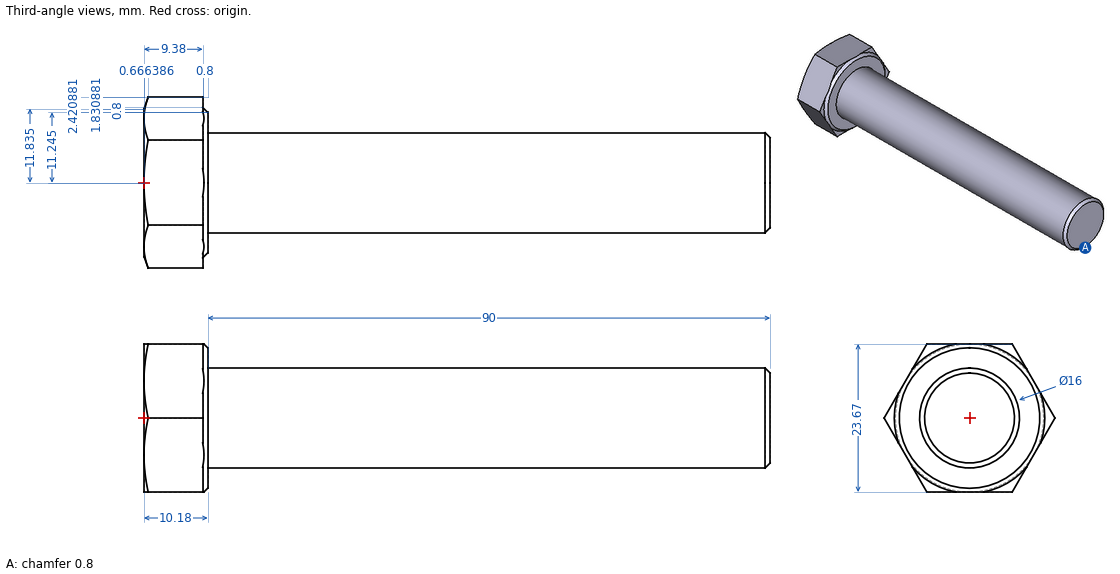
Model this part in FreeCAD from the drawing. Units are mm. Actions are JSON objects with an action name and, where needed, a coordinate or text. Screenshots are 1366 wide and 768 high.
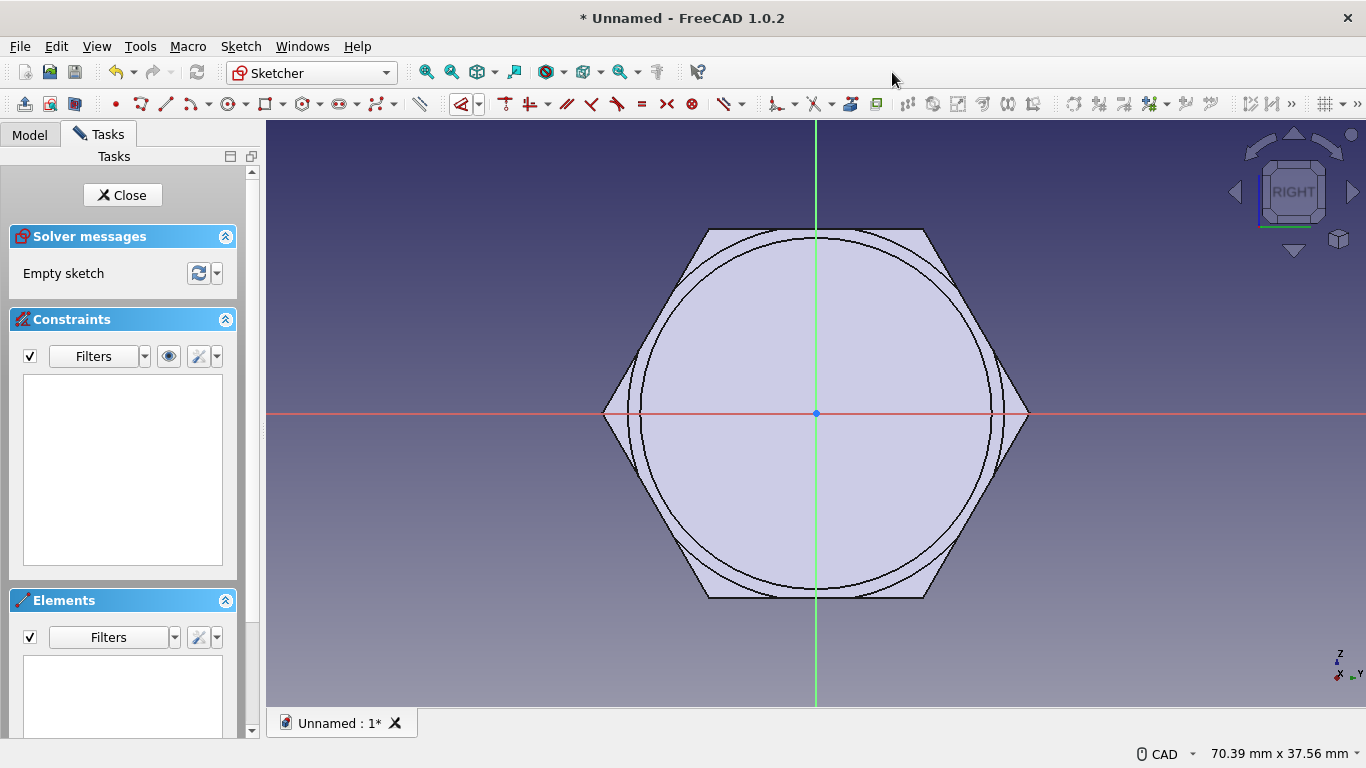
{"action": "scroll", "coordinate": [955, 413], "scroll_direction": "up", "scroll_amount": 2}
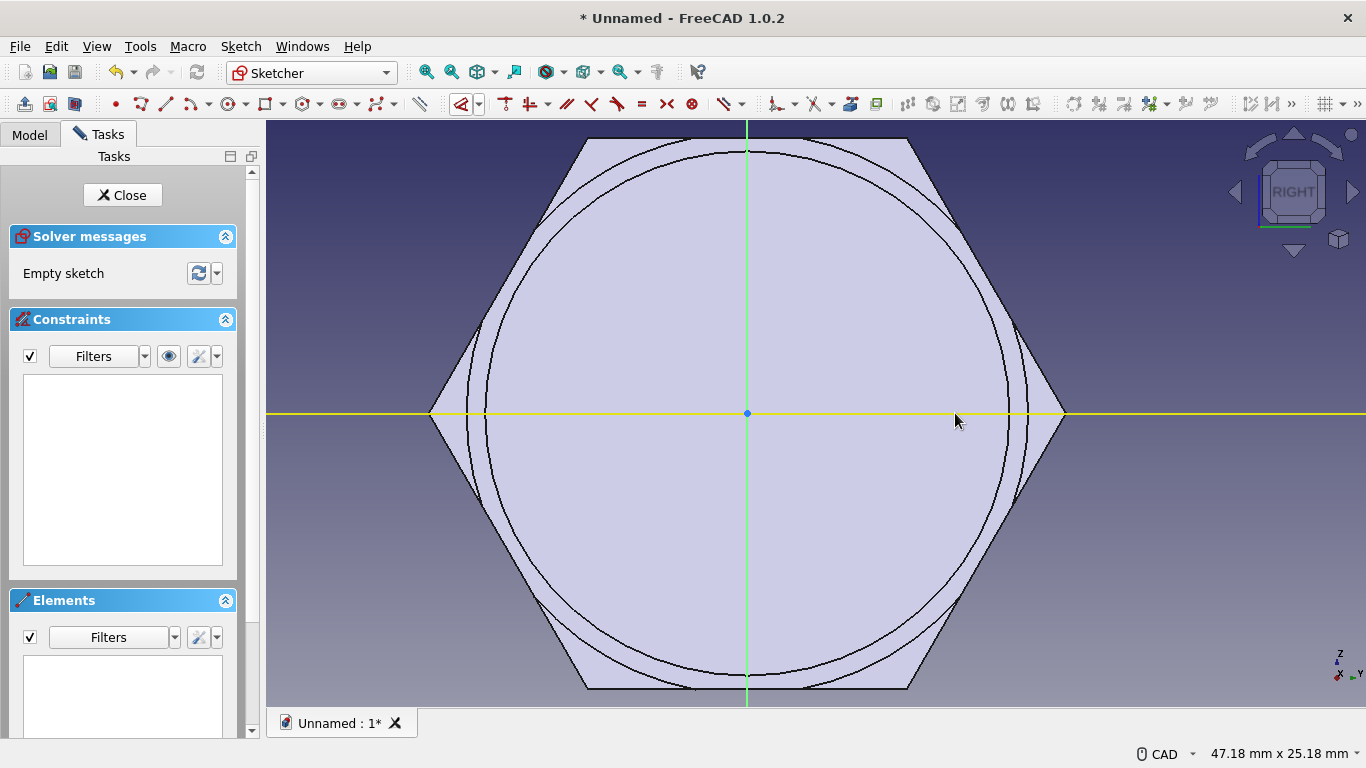
{"action": "key", "text": "g c"}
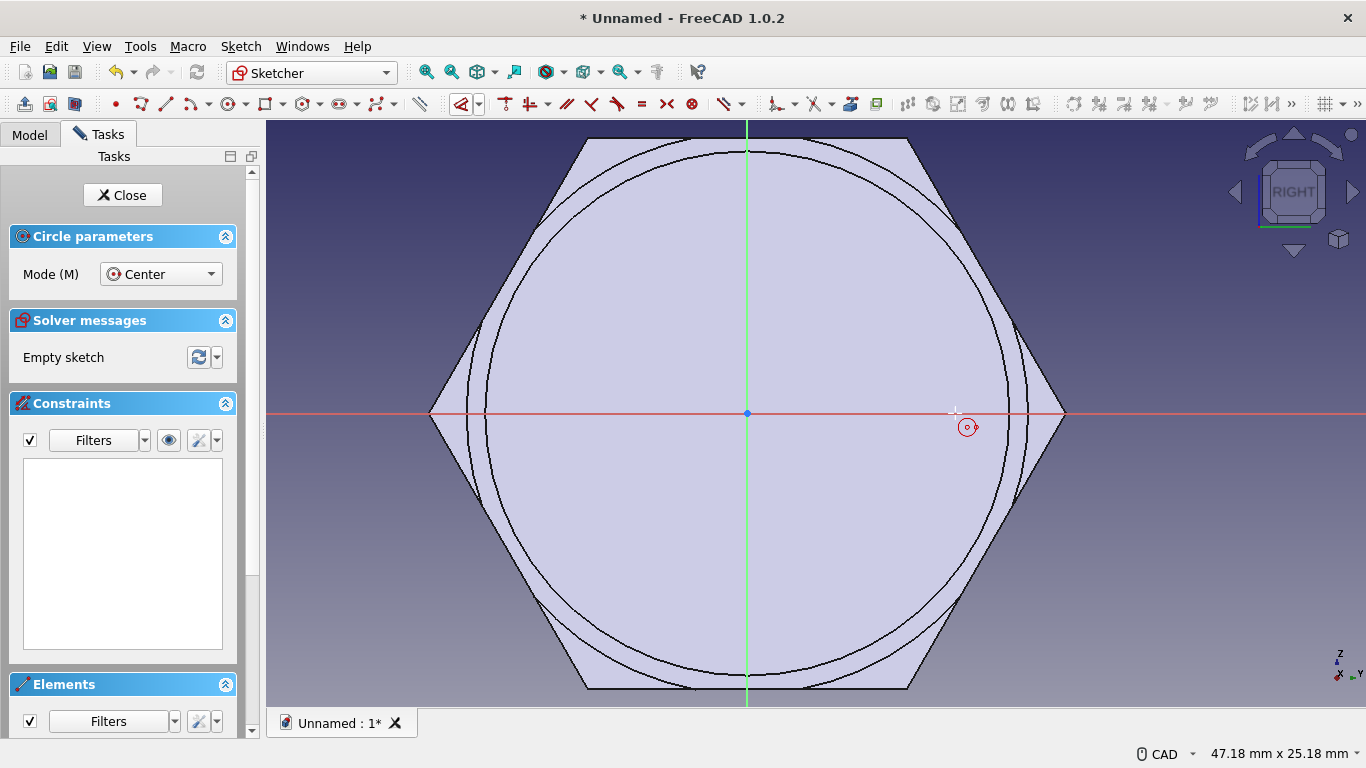
{"action": "left_click", "coordinate": [747, 413]}
{"action": "left_click", "coordinate": [879, 282]}
{"action": "key", "text": "Escape"}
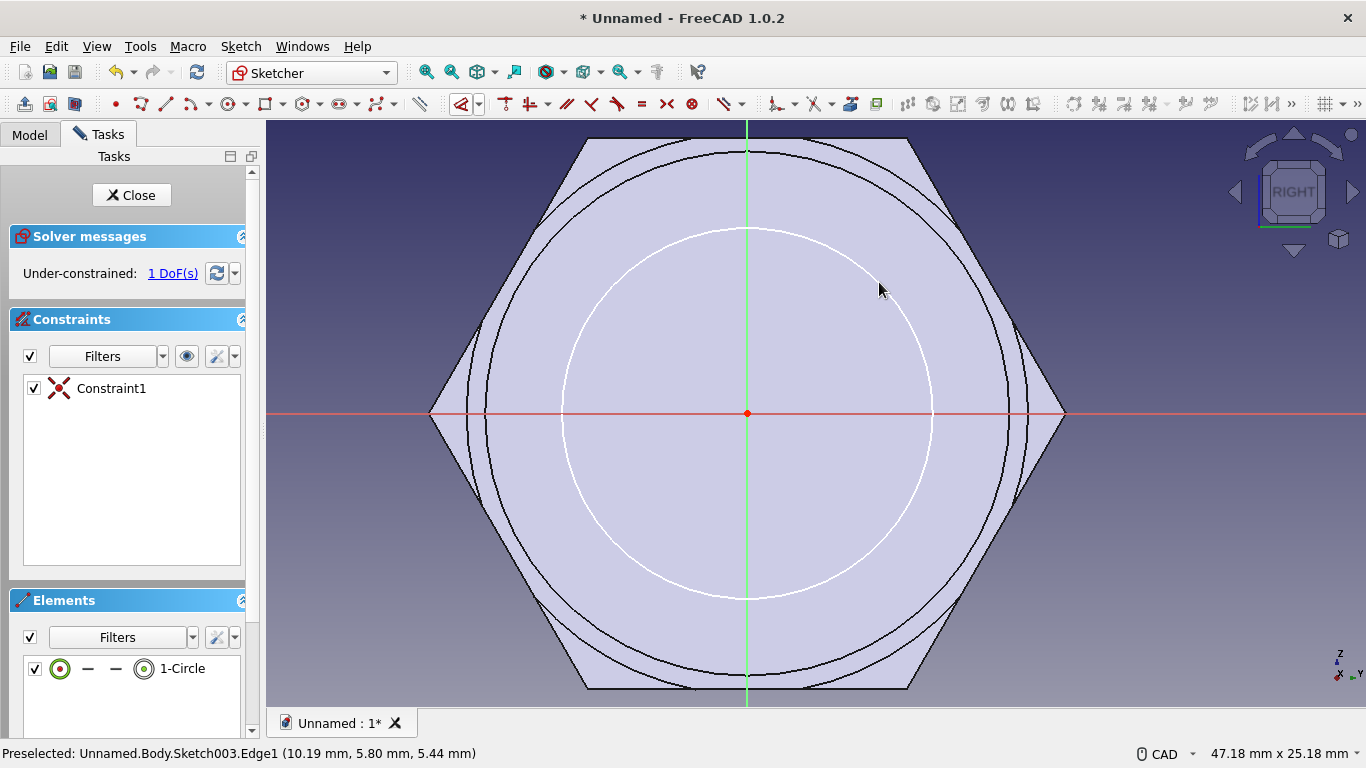
{"action": "left_click", "coordinate": [878, 282]}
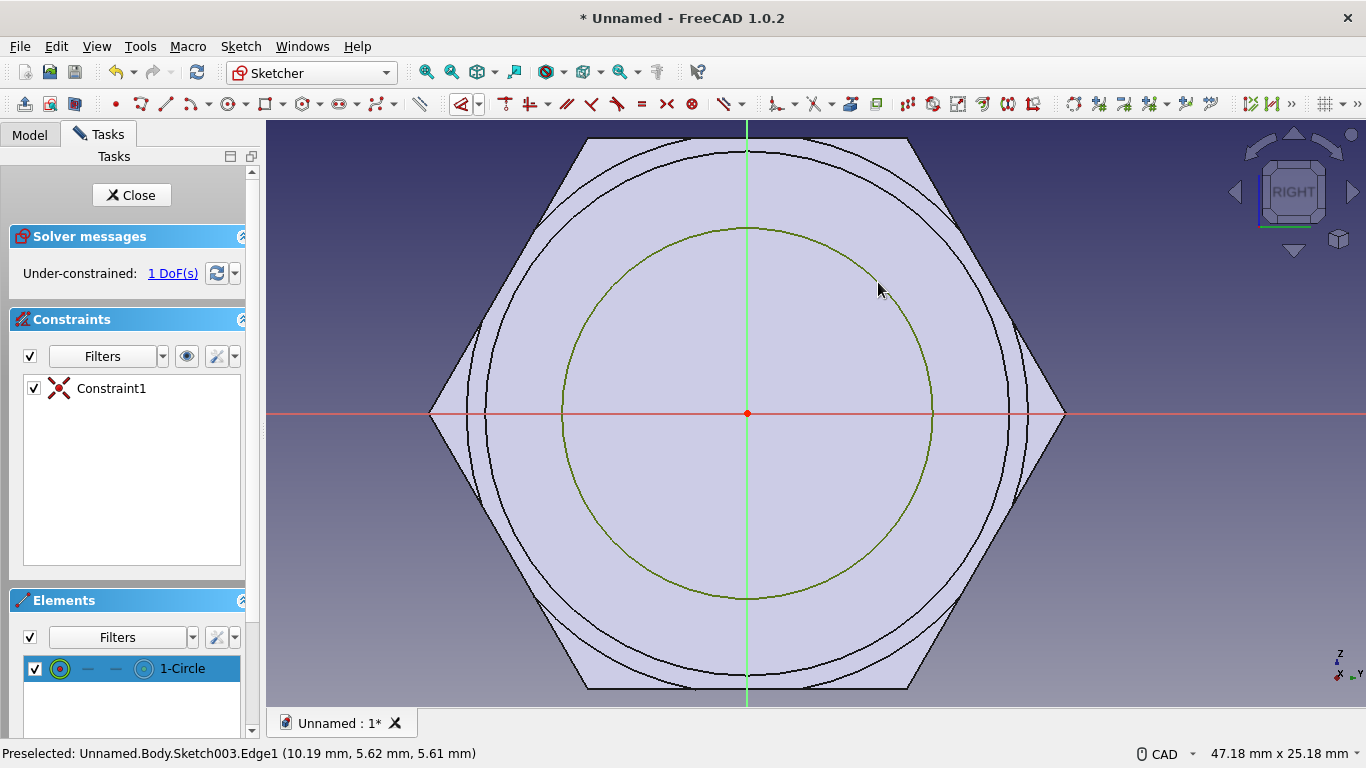
{"action": "key", "text": "k o"}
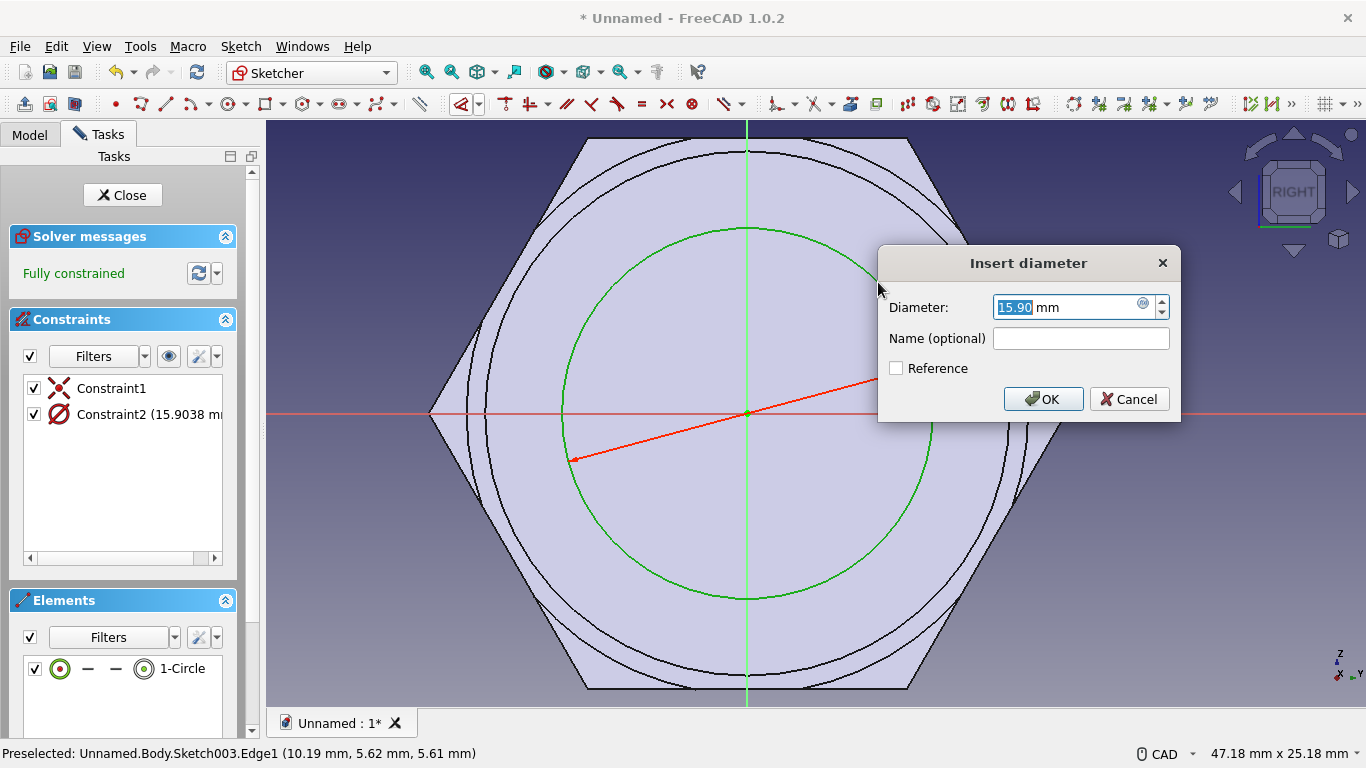
{"action": "type", "text": "16"}
{"action": "key", "text": "Return"}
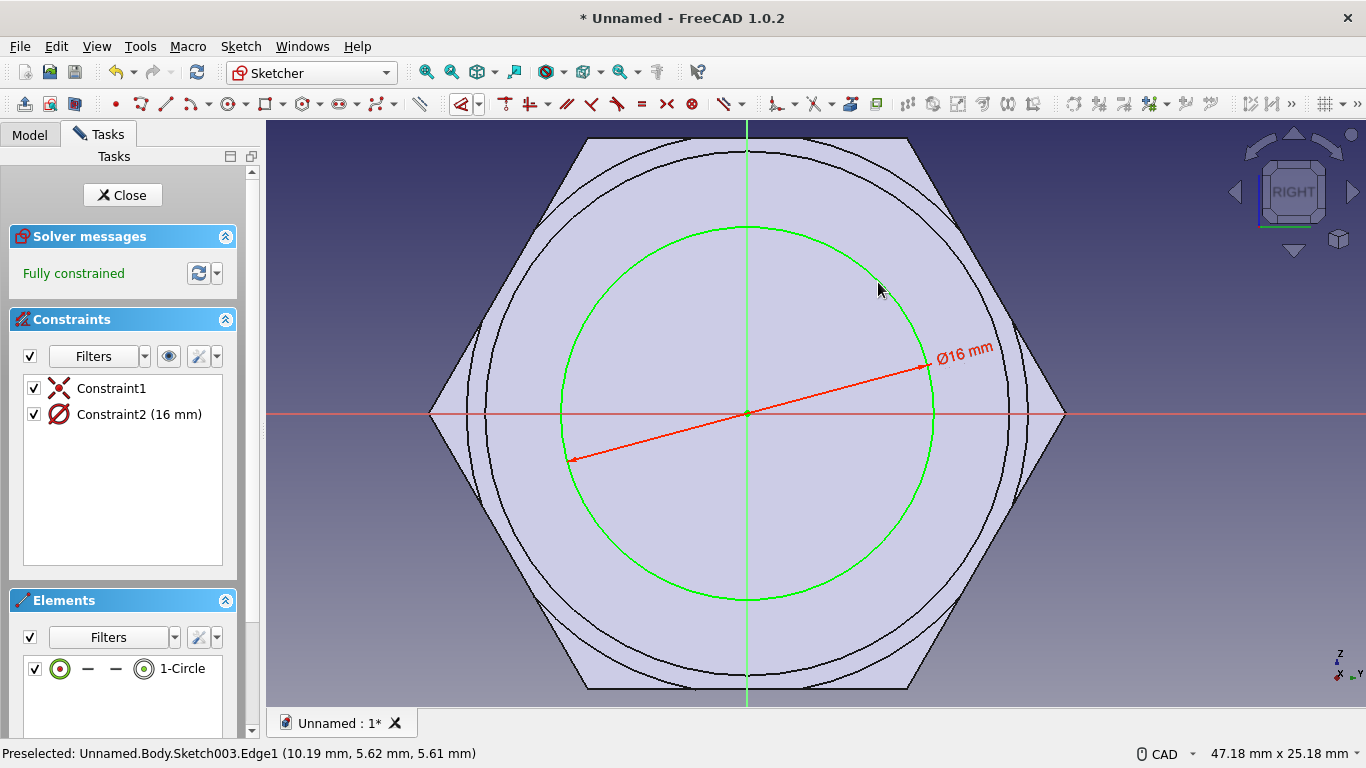
{"action": "left_click", "coordinate": [123, 195]}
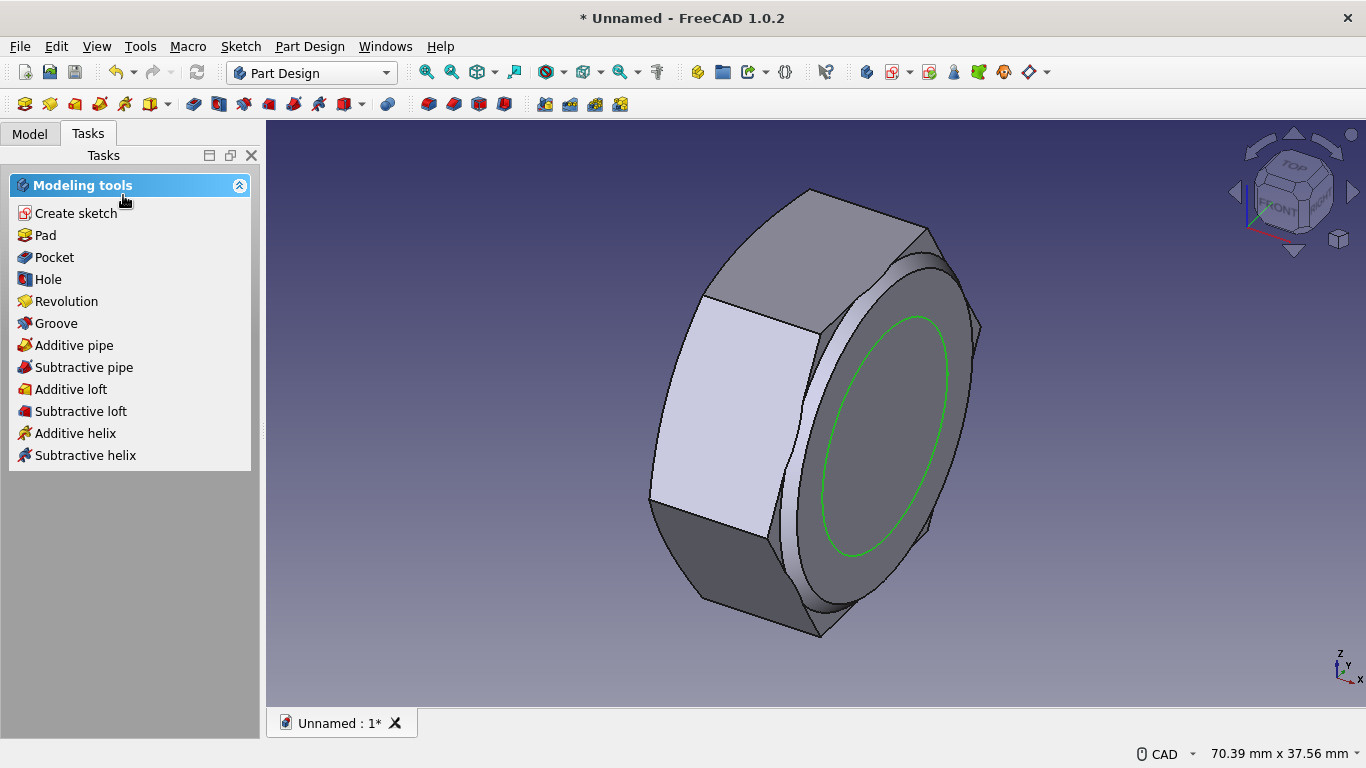
{"action": "left_click", "coordinate": [25, 104]}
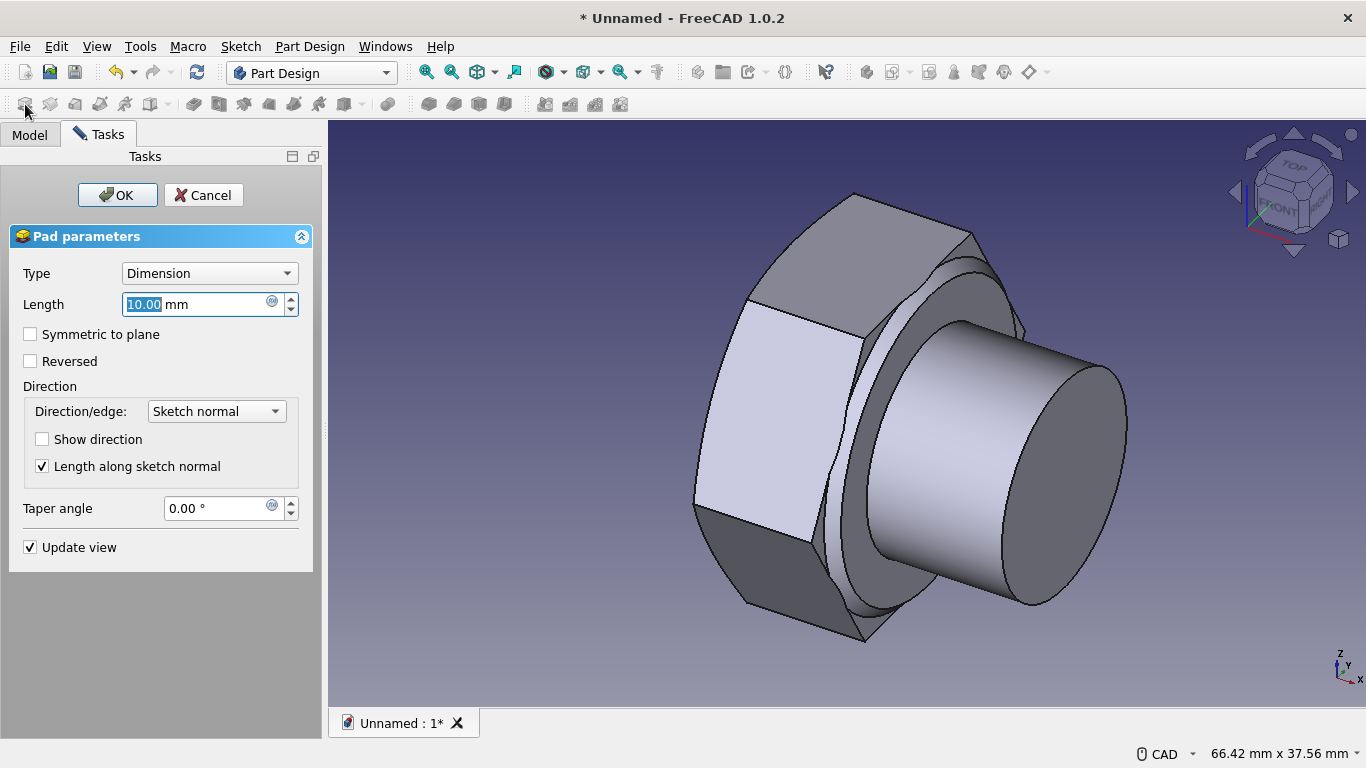
{"action": "type", "text": "90"}
{"action": "key", "text": "Tab"}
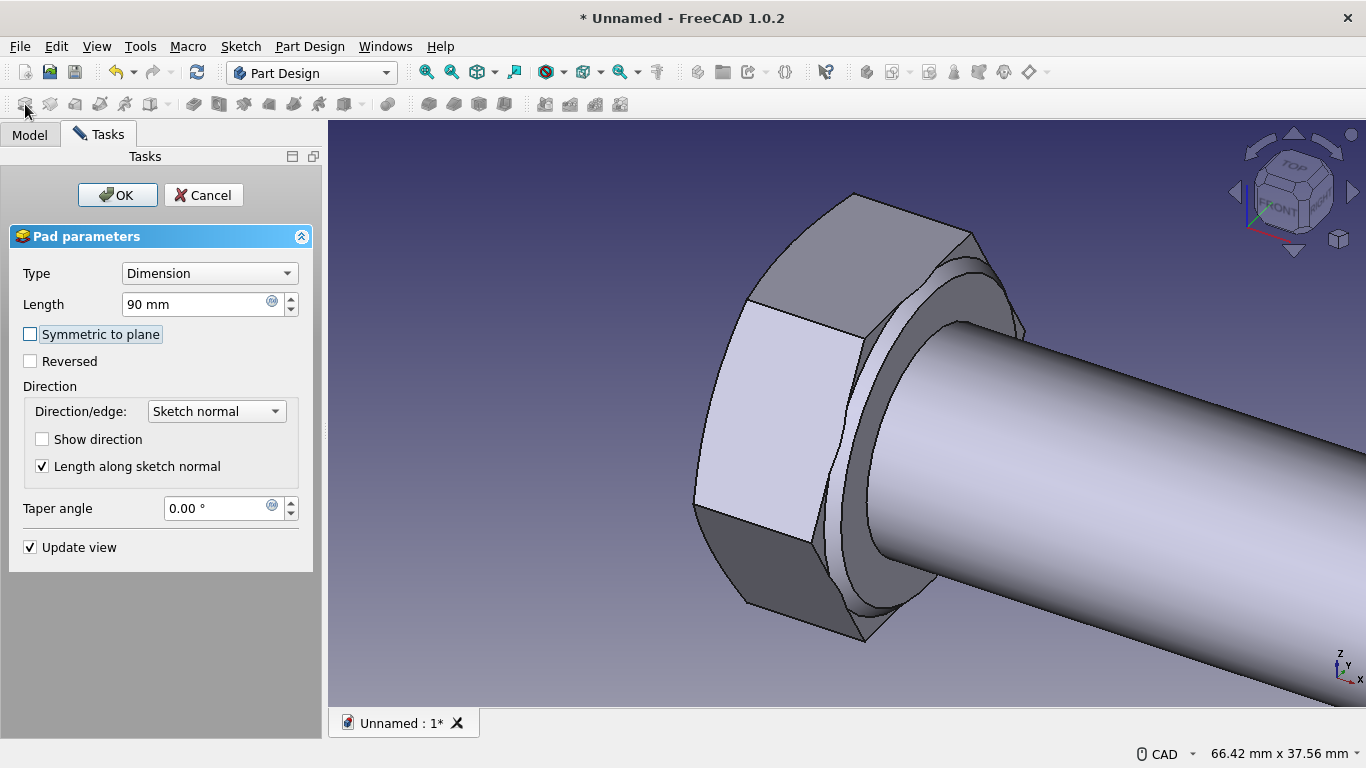
{"action": "left_click", "coordinate": [118, 195]}